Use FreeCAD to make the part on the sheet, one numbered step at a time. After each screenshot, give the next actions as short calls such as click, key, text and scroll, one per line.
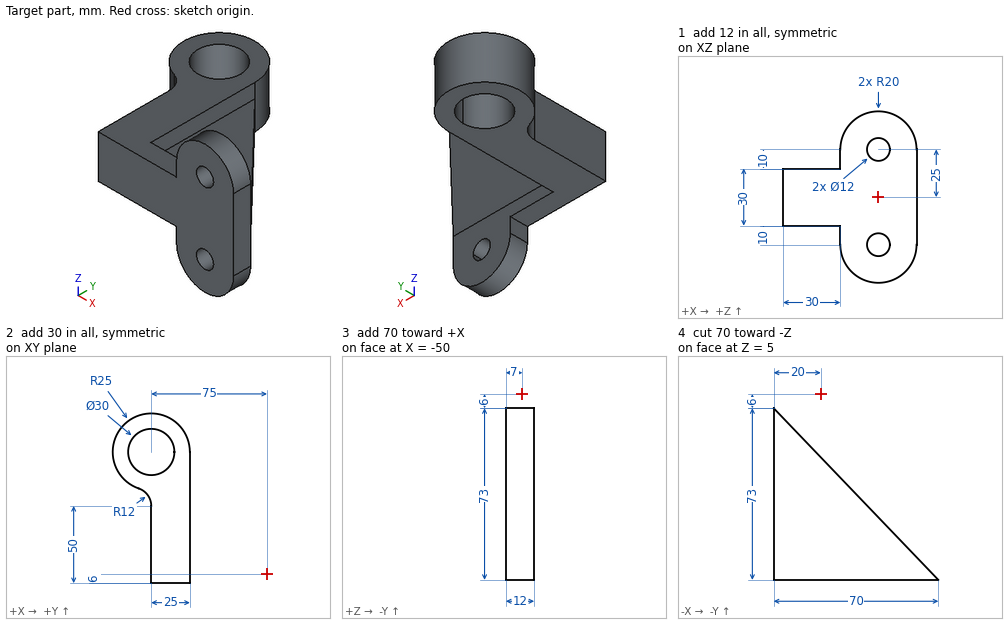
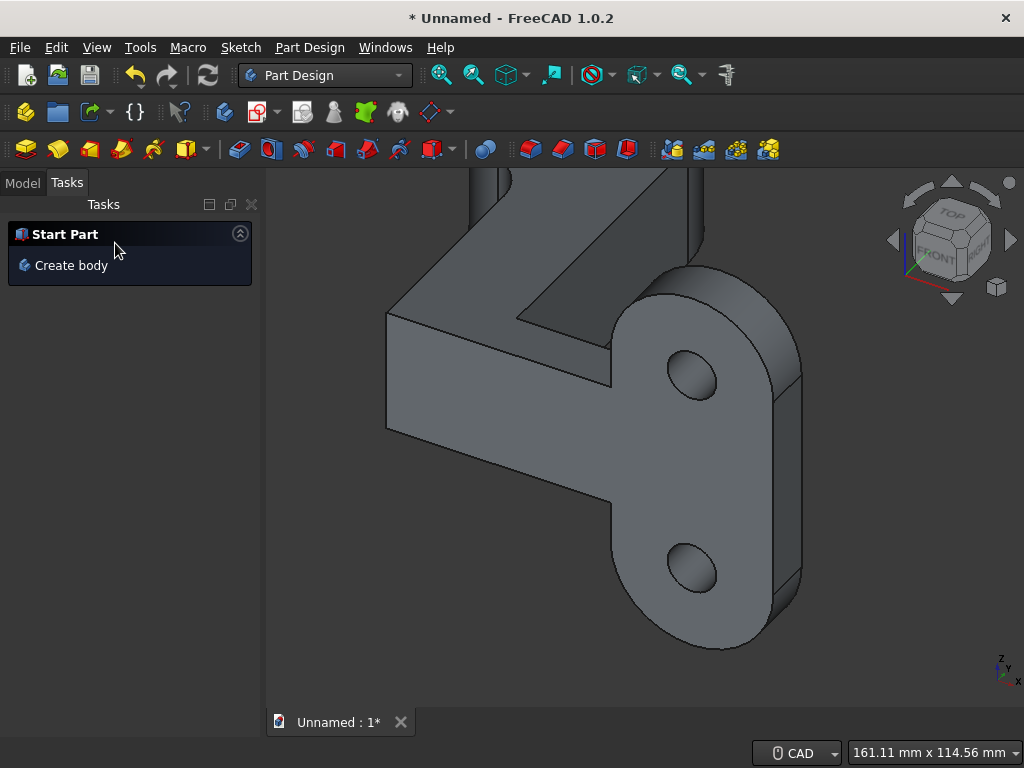
click(442, 76)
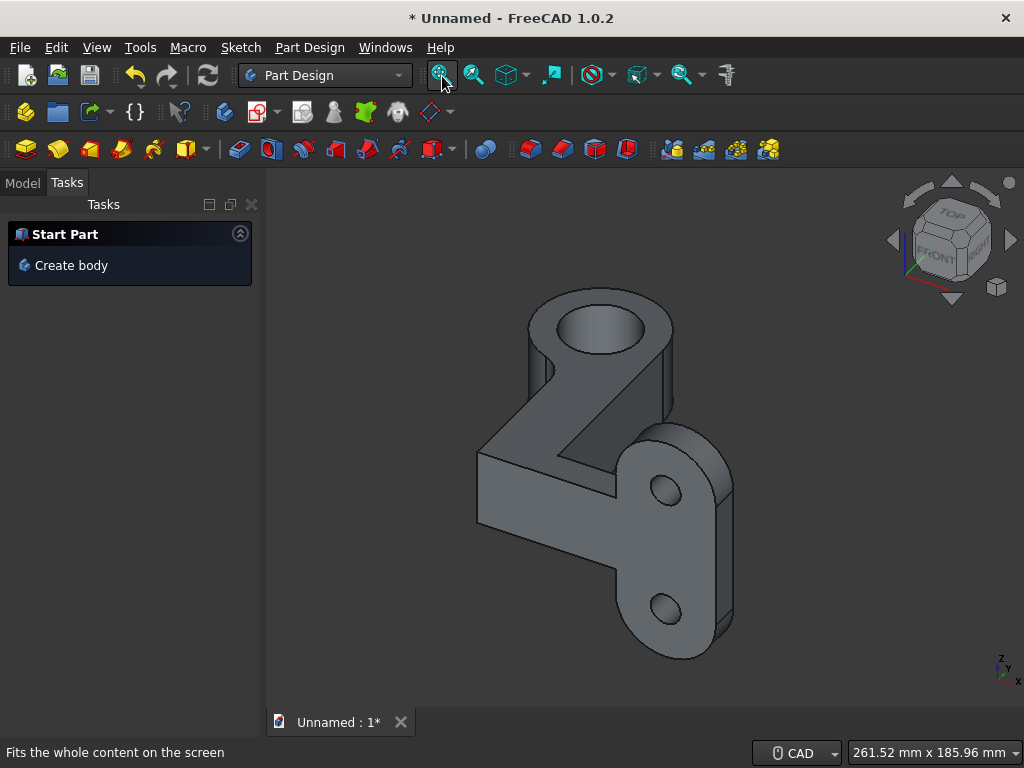
click(626, 422)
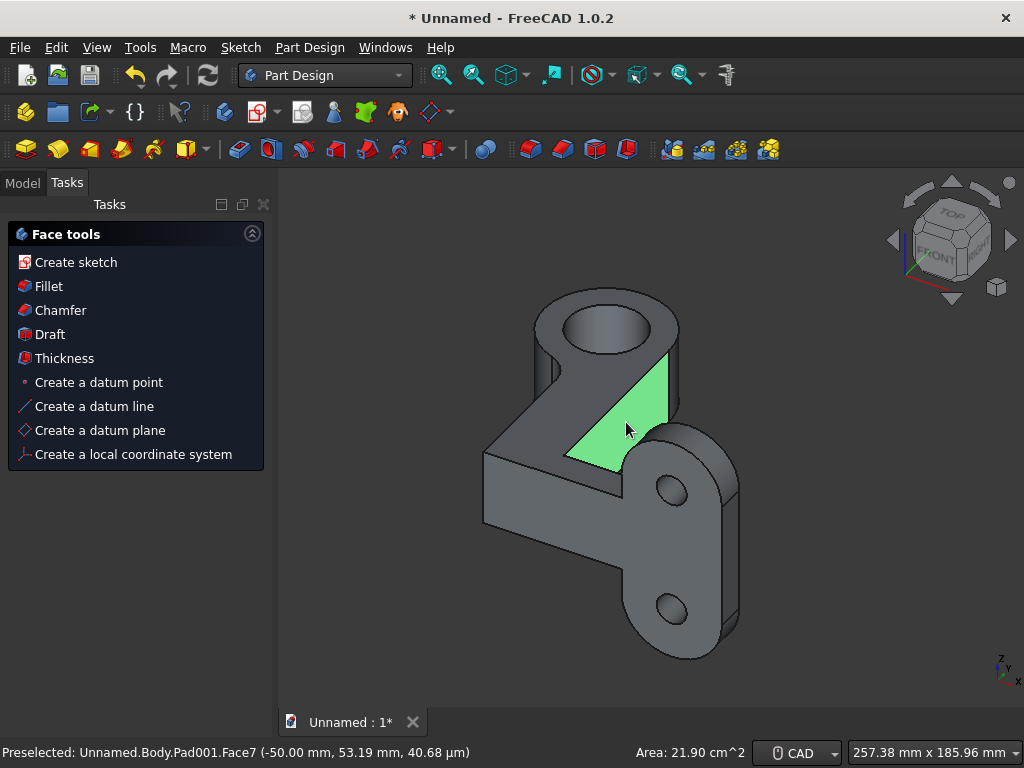
click(258, 112)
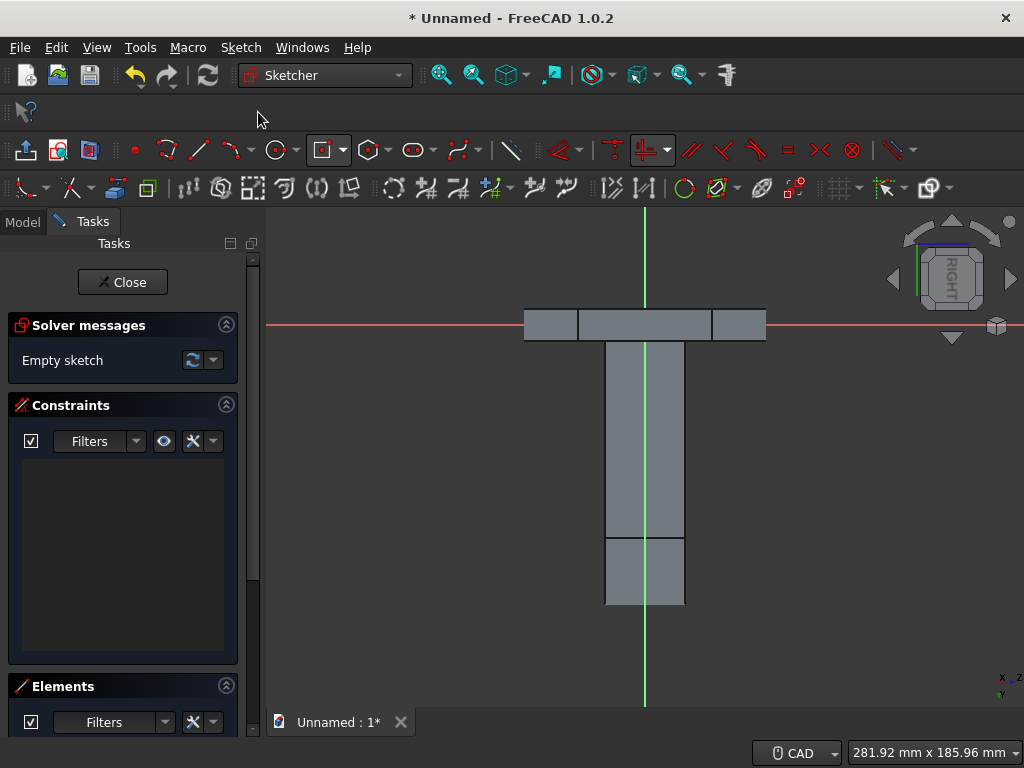
scroll(776, 380, up, 2)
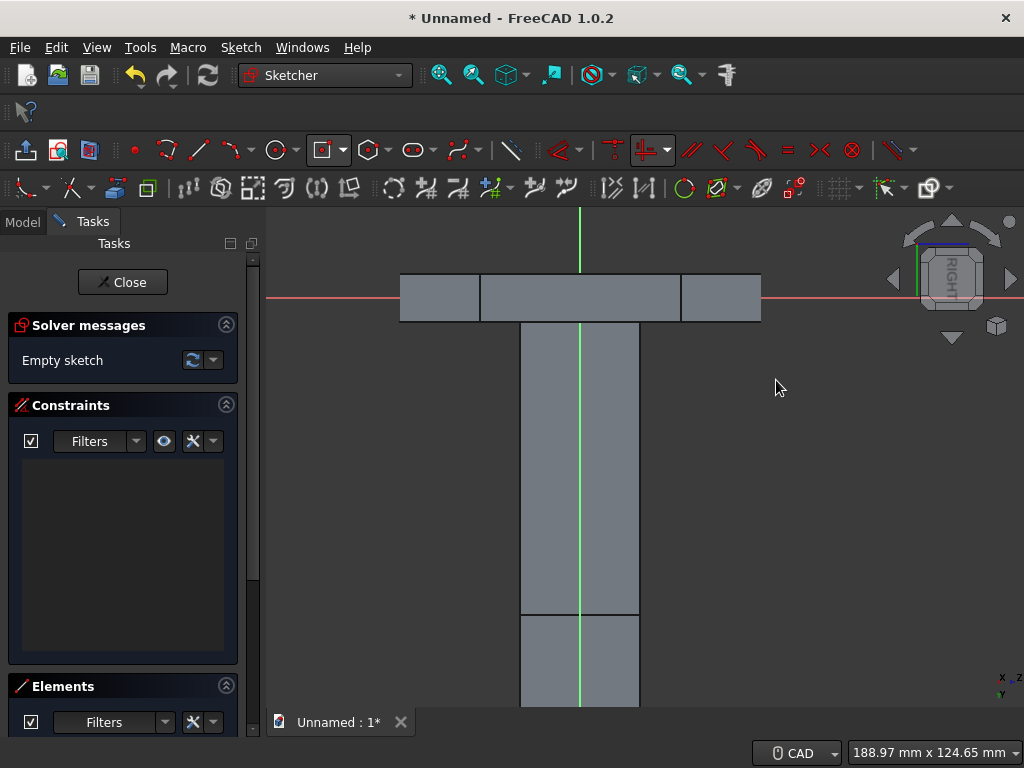
key(g)
key(r)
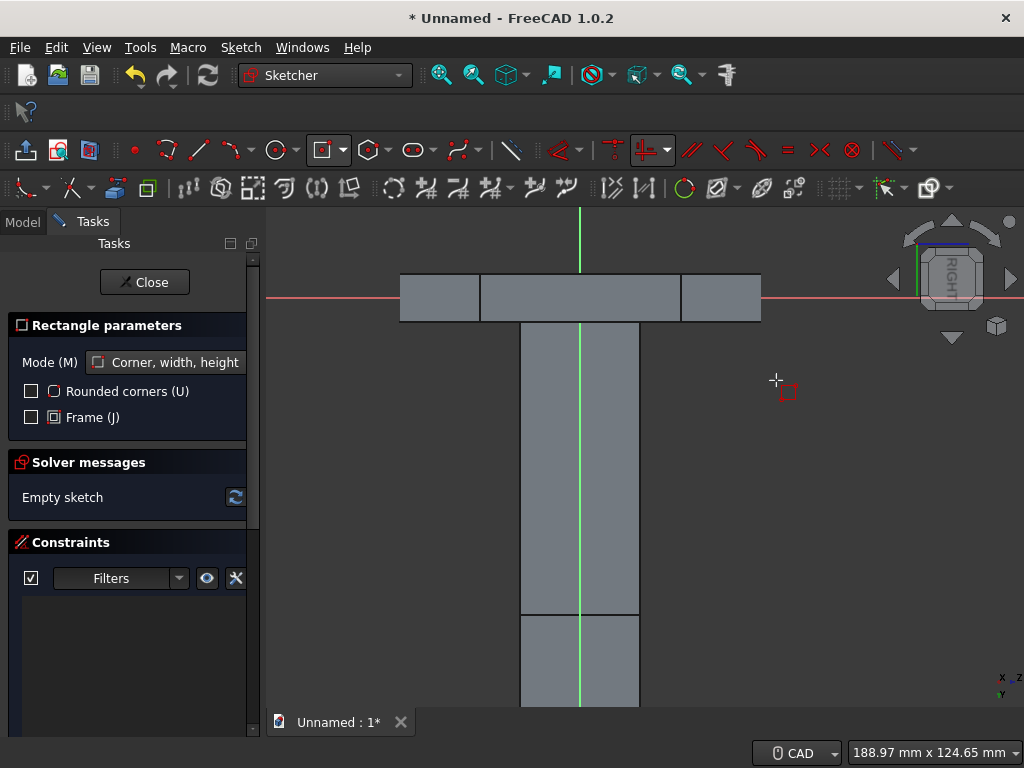
click(552, 322)
click(600, 615)
key(Escape)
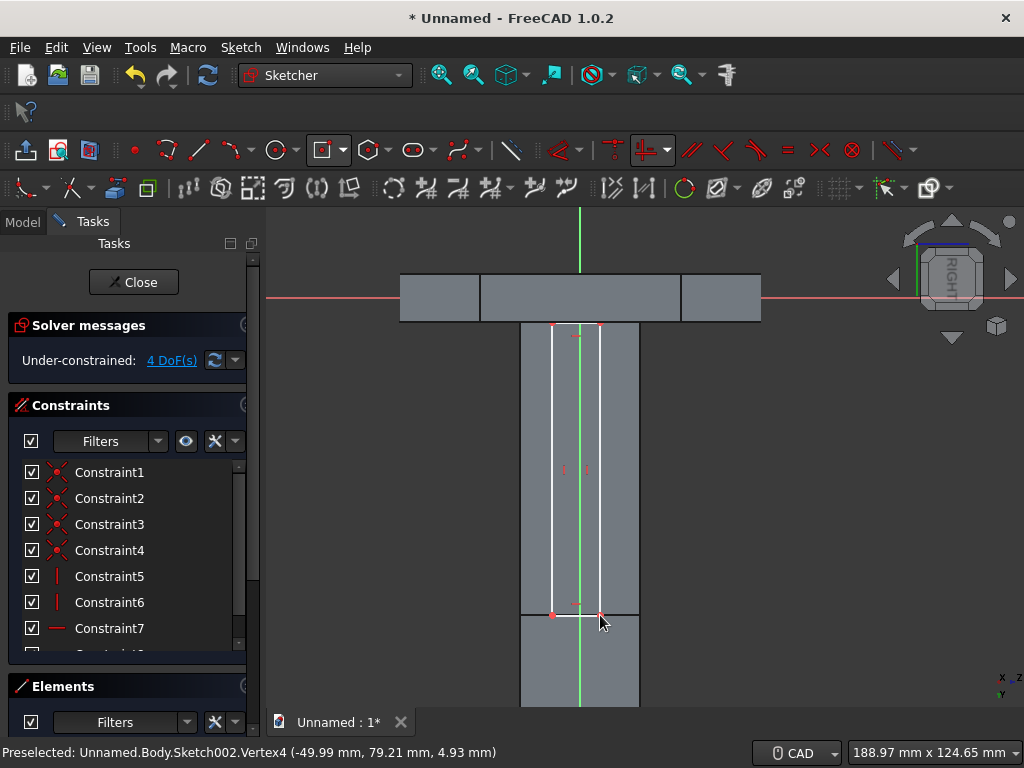
click(558, 150)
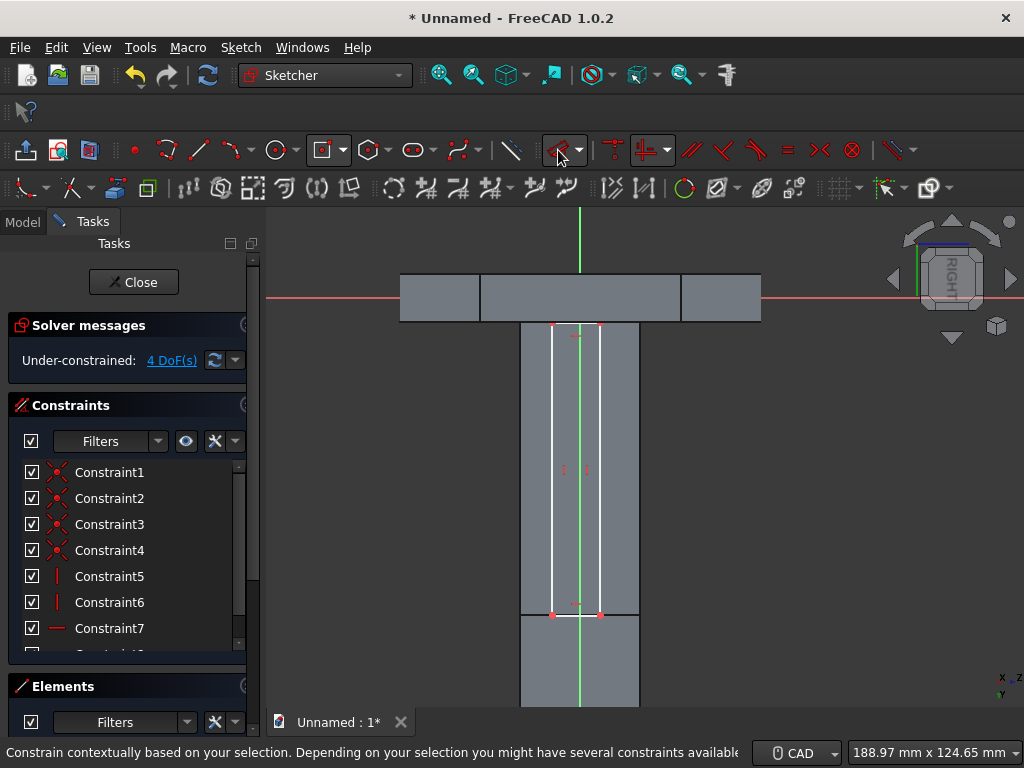
click(552, 411)
click(518, 470)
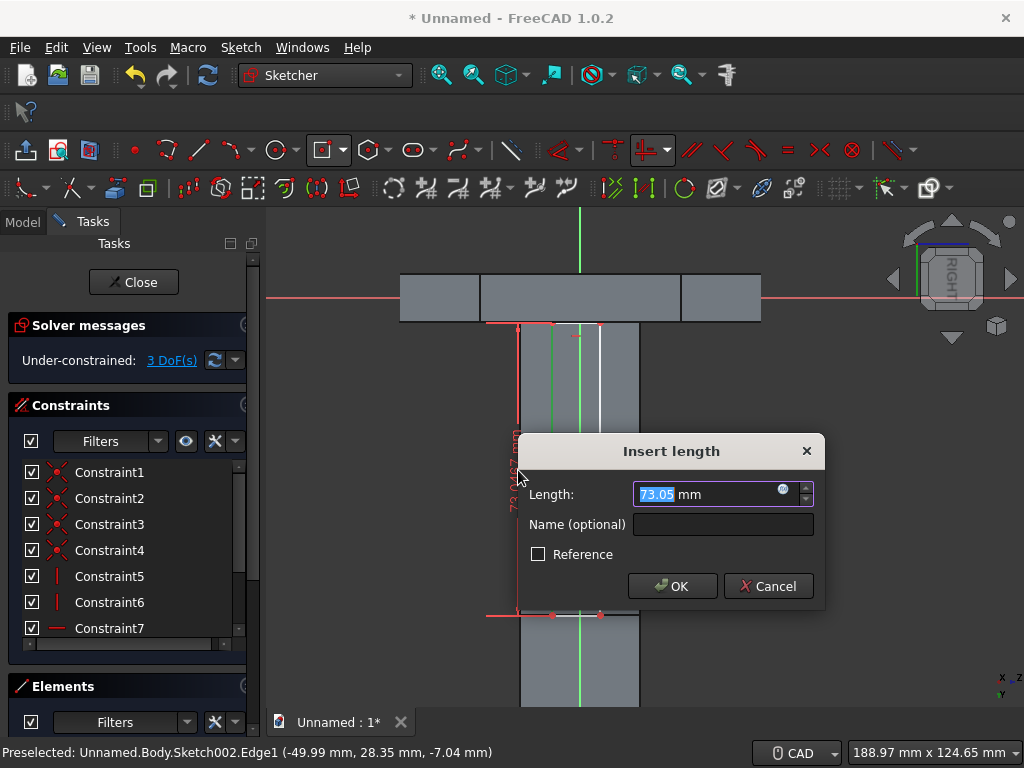
text(73)
key(Return)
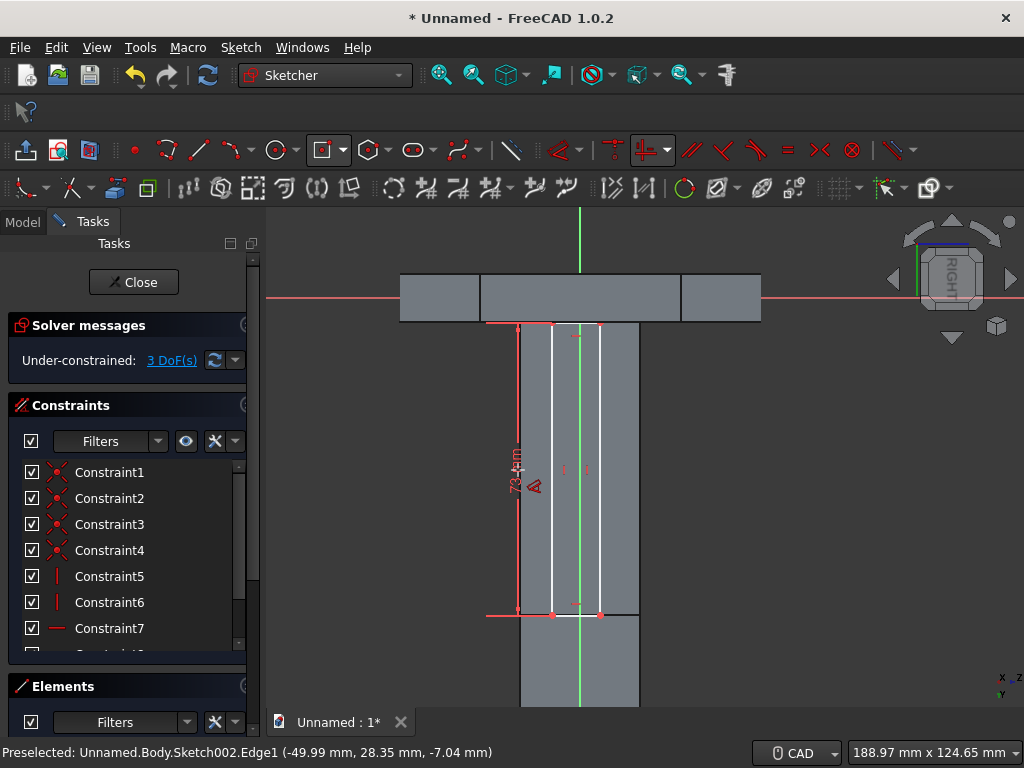
click(566, 616)
click(565, 650)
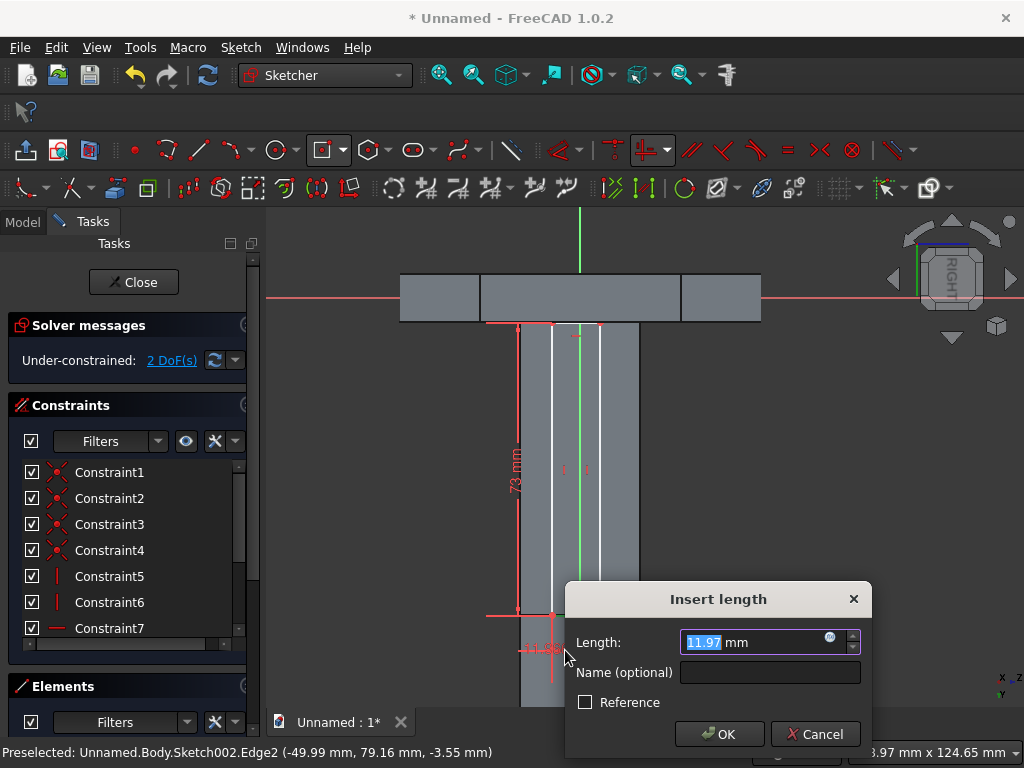
text(12)
key(Return)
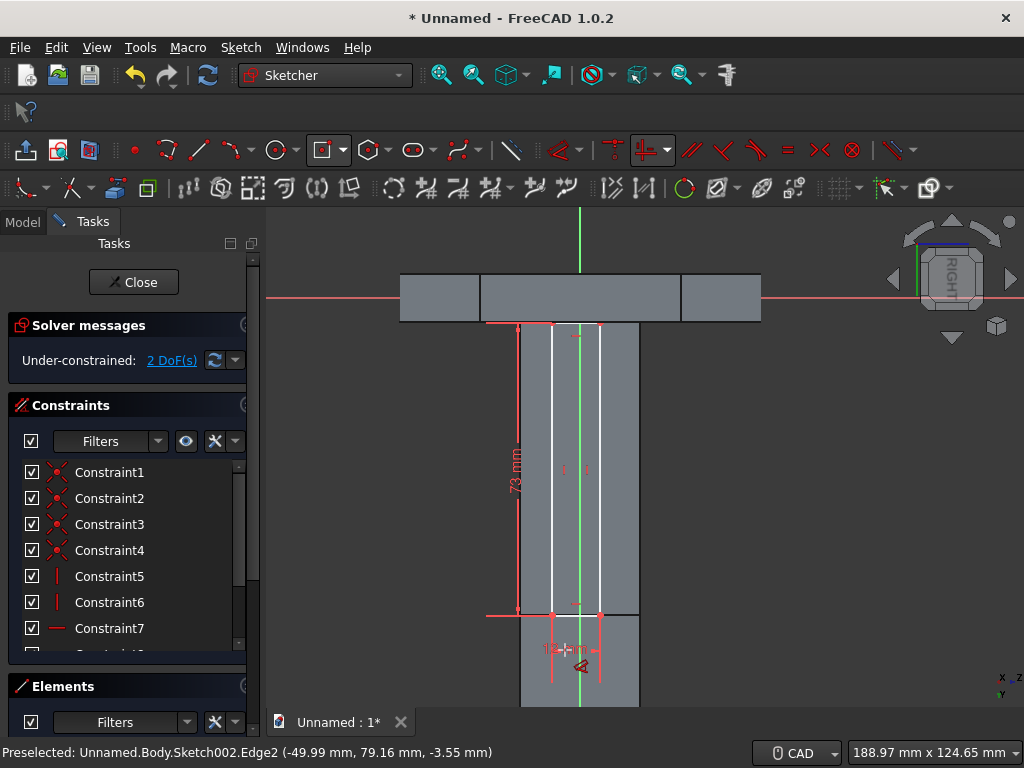
scroll(552, 323, up, 2)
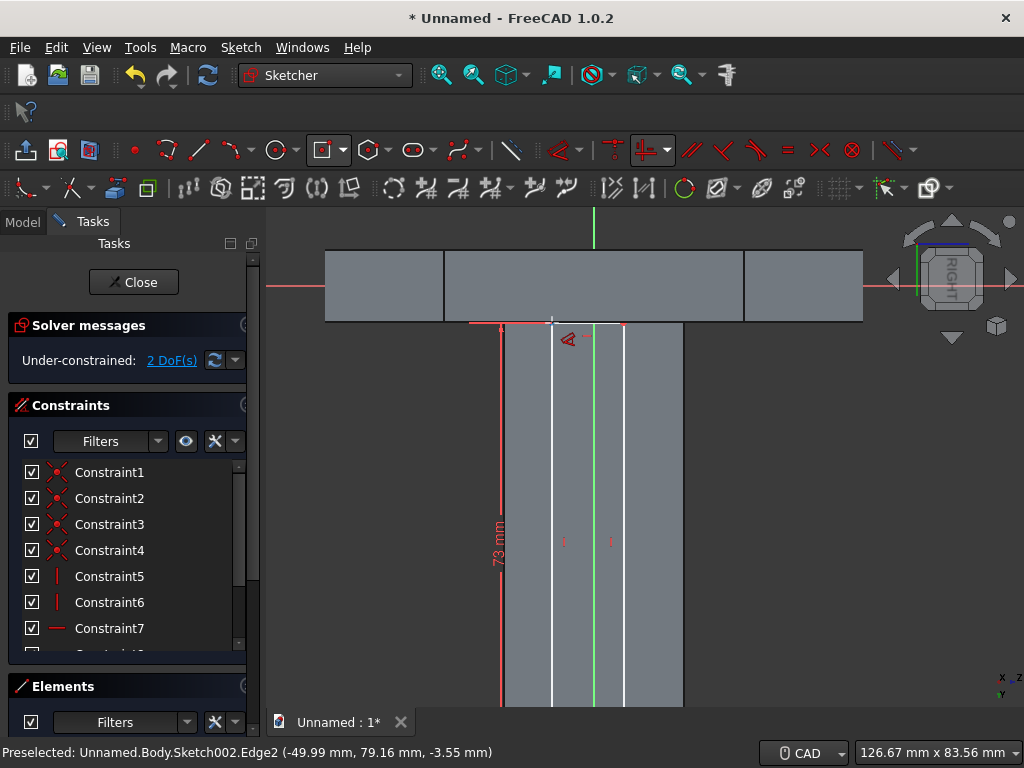
click(552, 323)
click(573, 252)